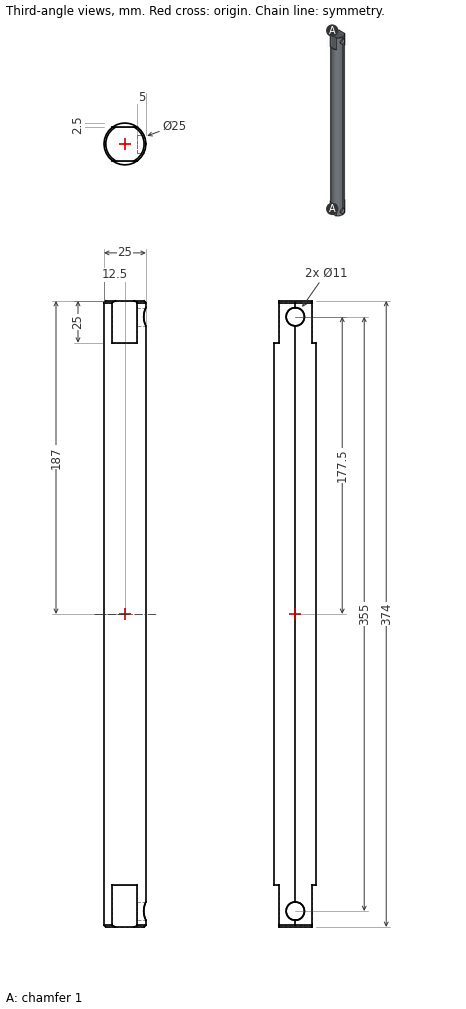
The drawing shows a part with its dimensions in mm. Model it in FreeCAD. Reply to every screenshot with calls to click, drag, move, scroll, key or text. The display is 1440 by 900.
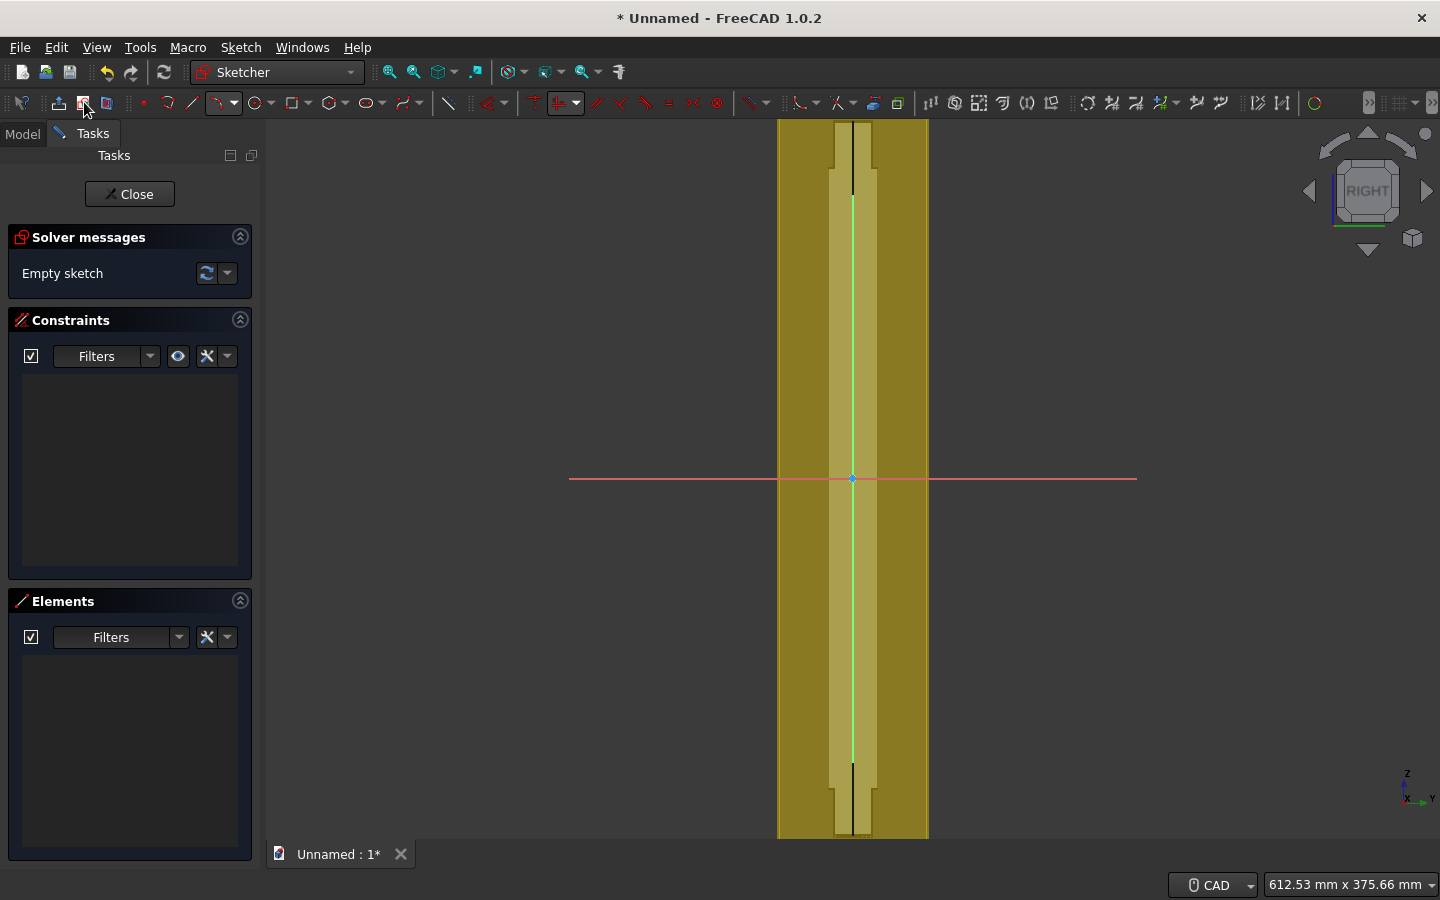
scroll(645, 479, down, 2)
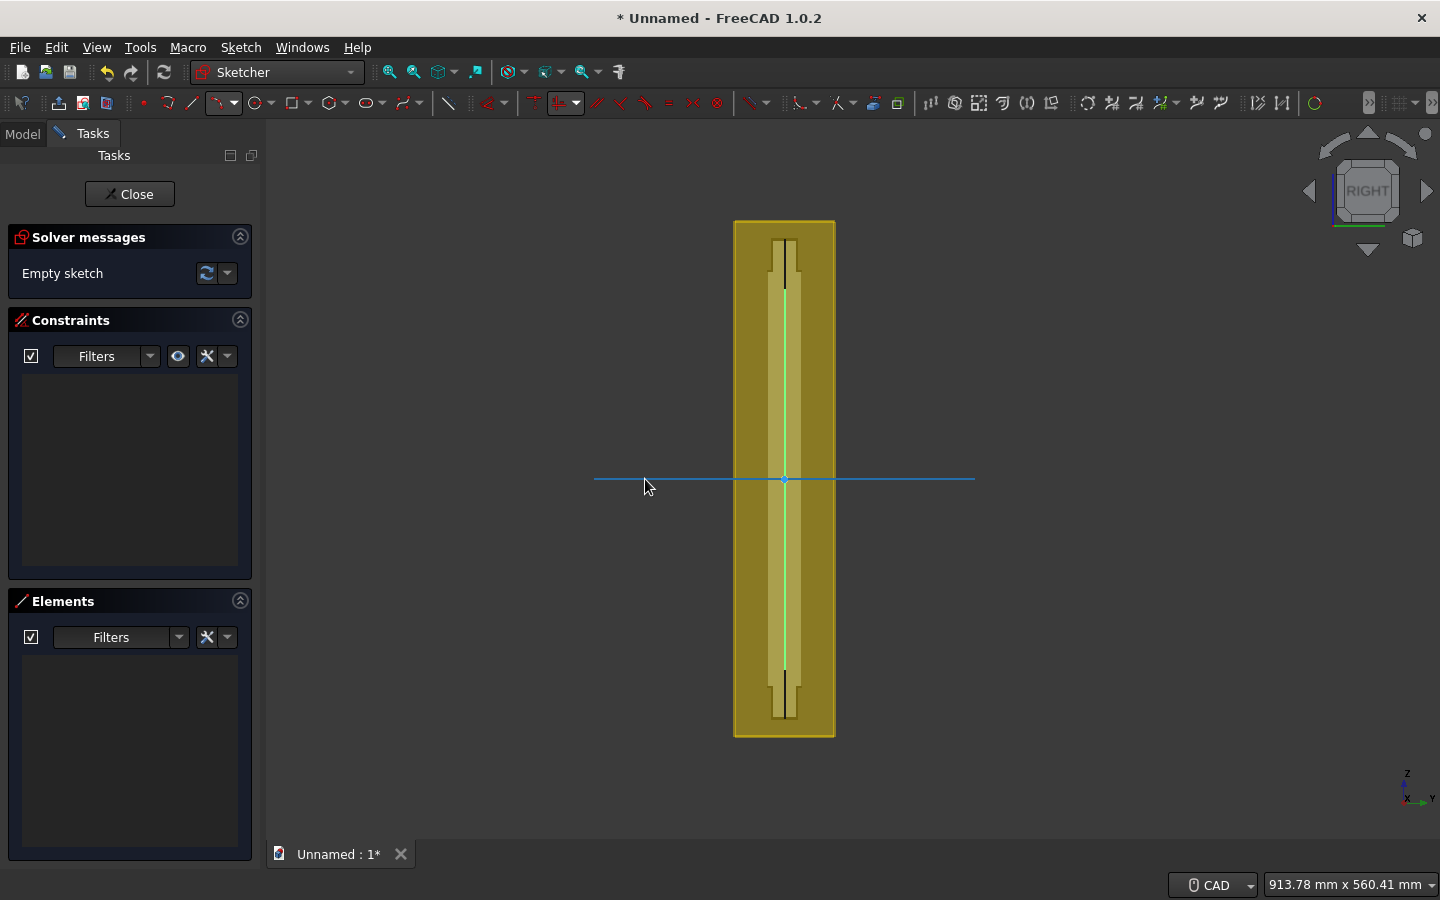
click(256, 104)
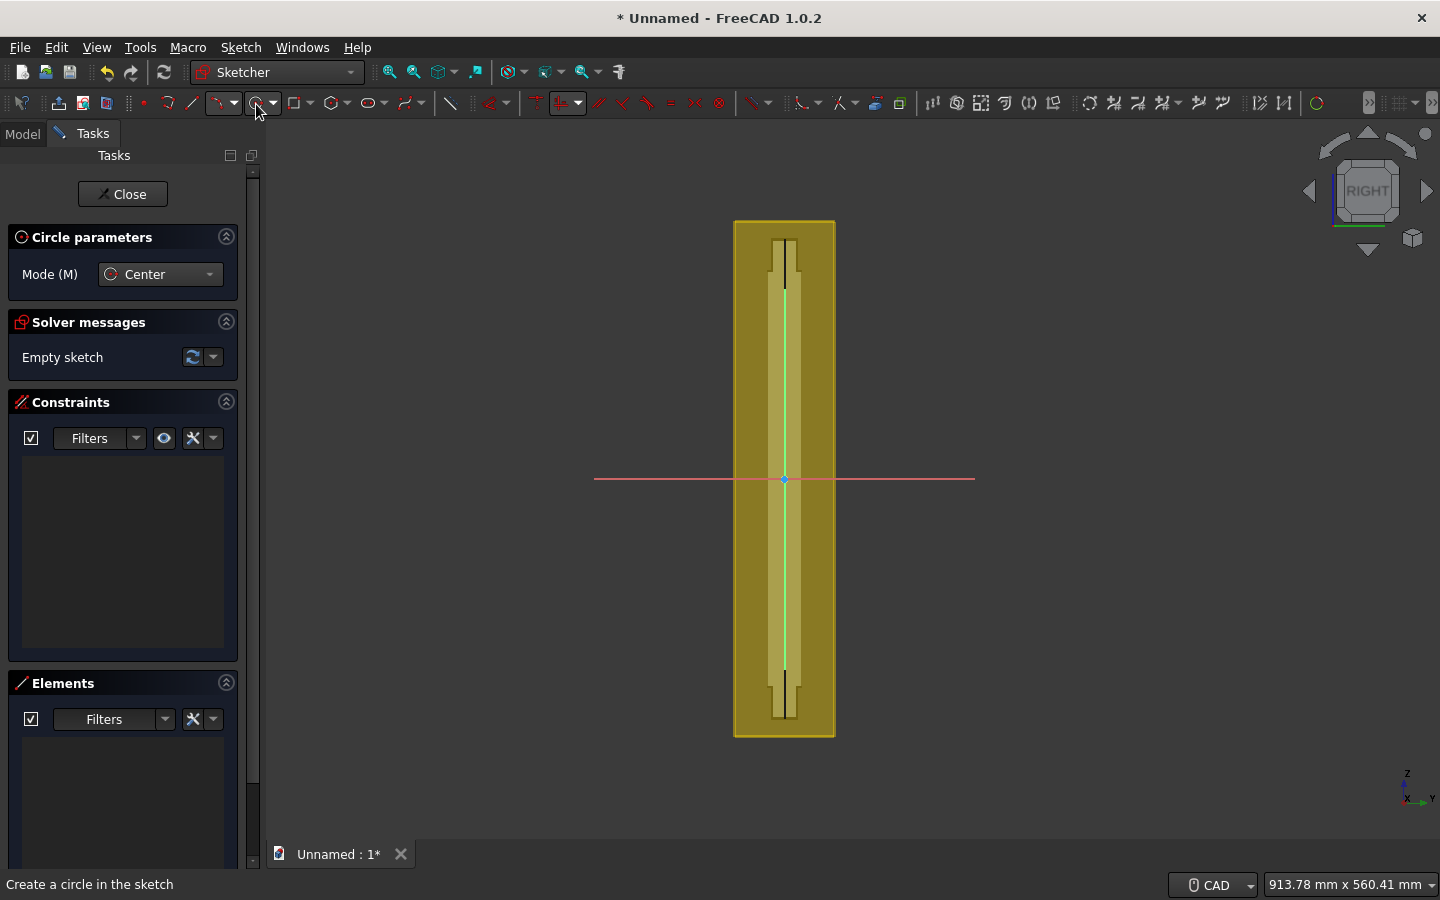
scroll(785, 251, up, 6)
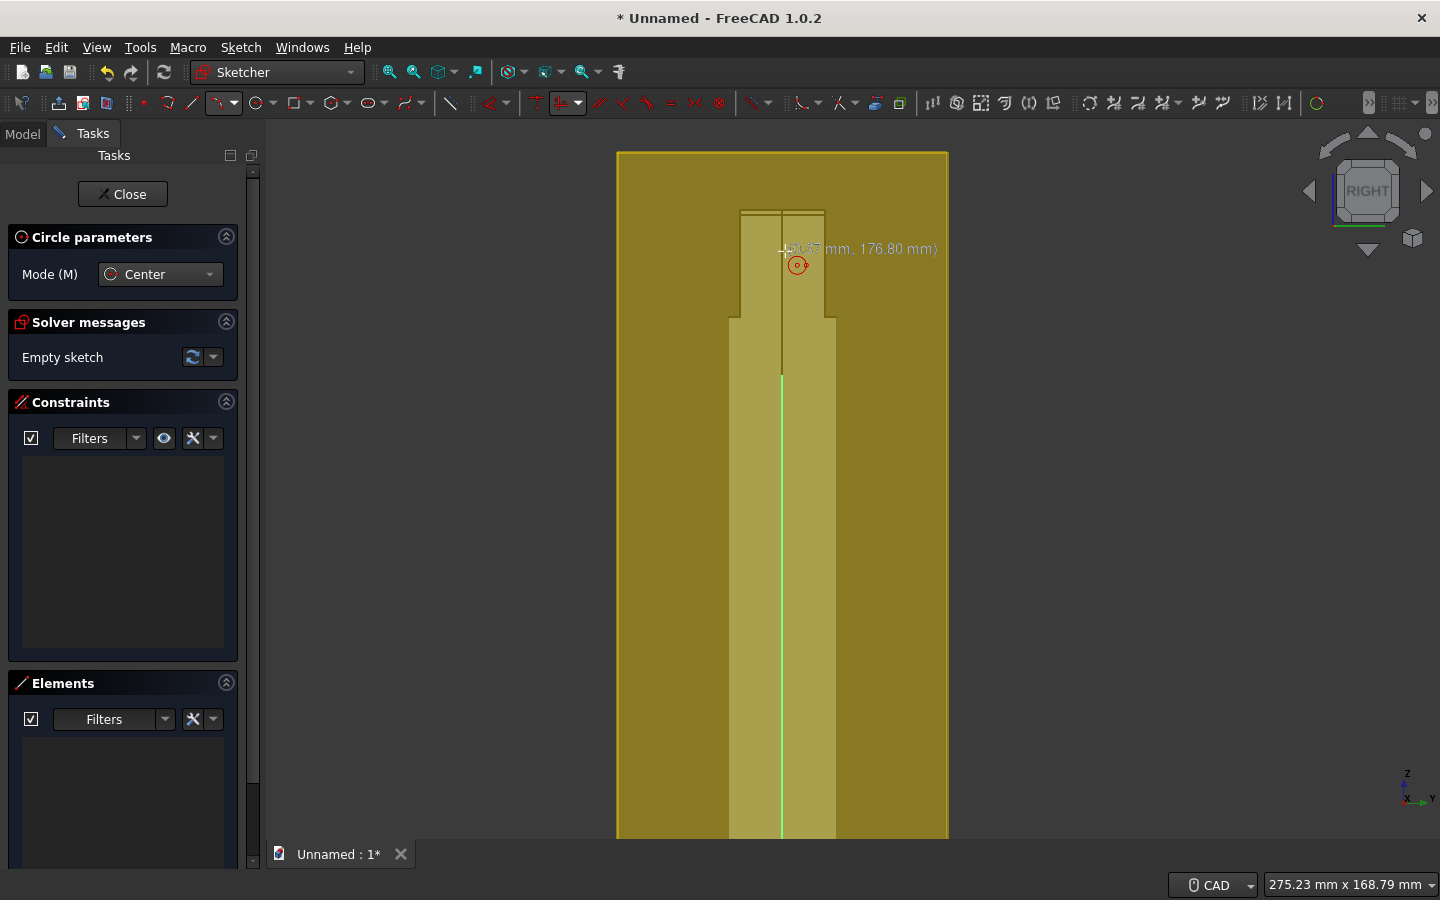
click(782, 251)
click(799, 234)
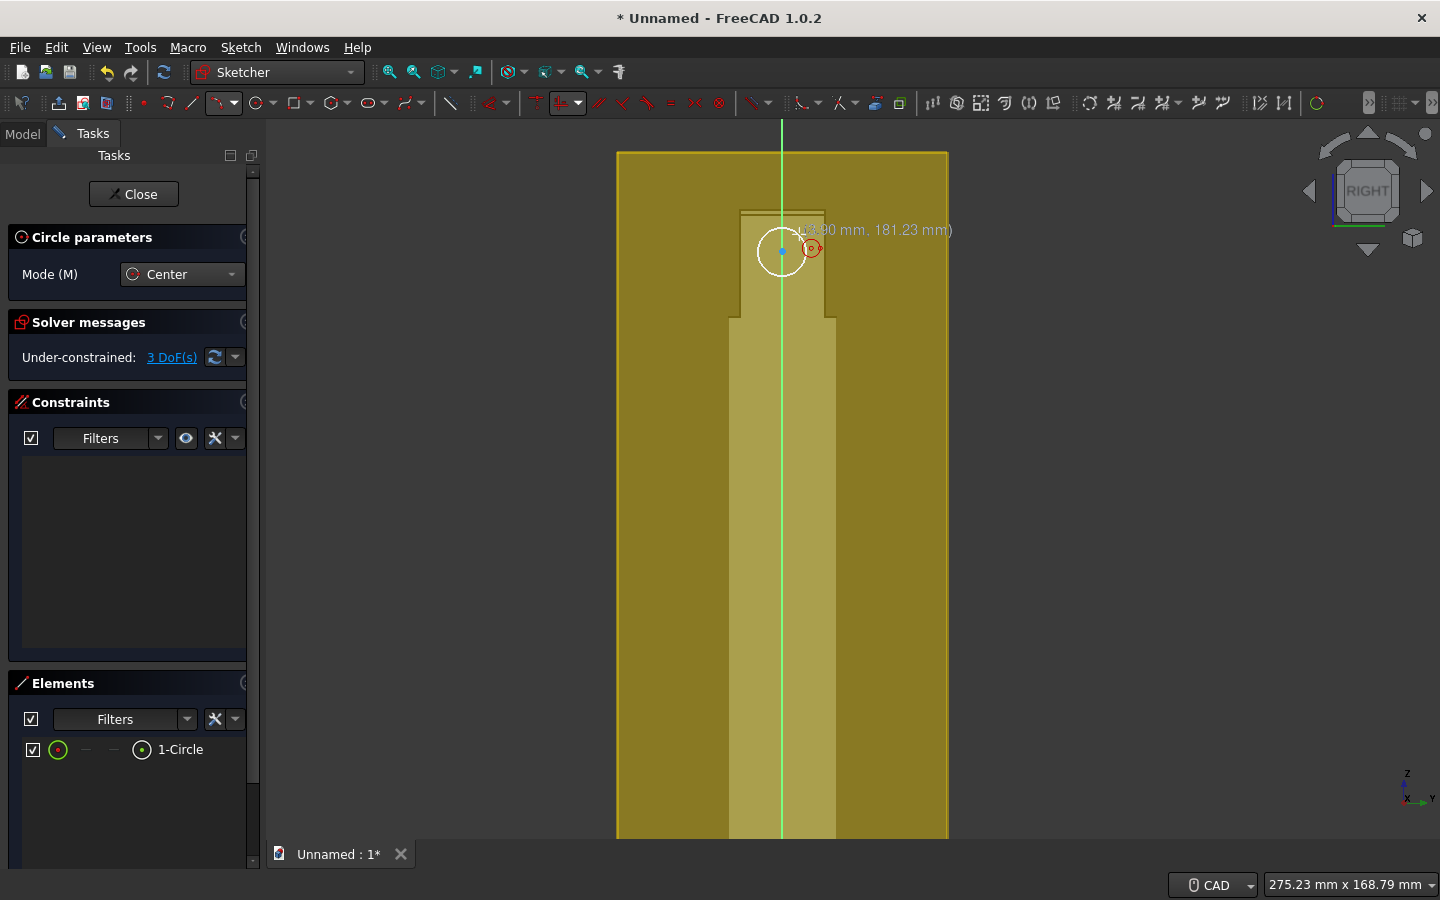
scroll(785, 251, down, 6)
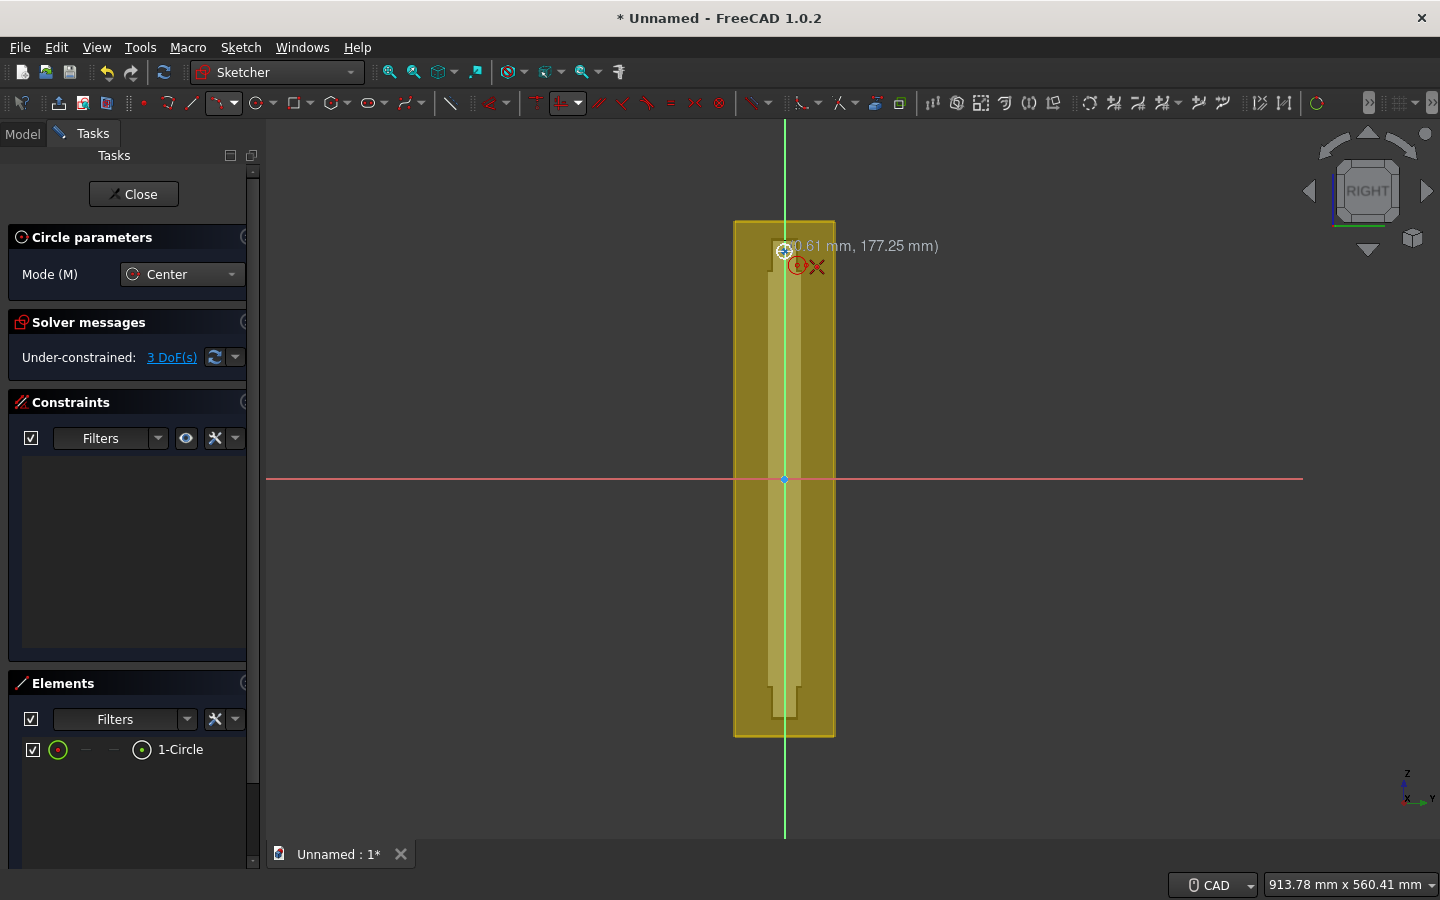
scroll(785, 707, up, 6)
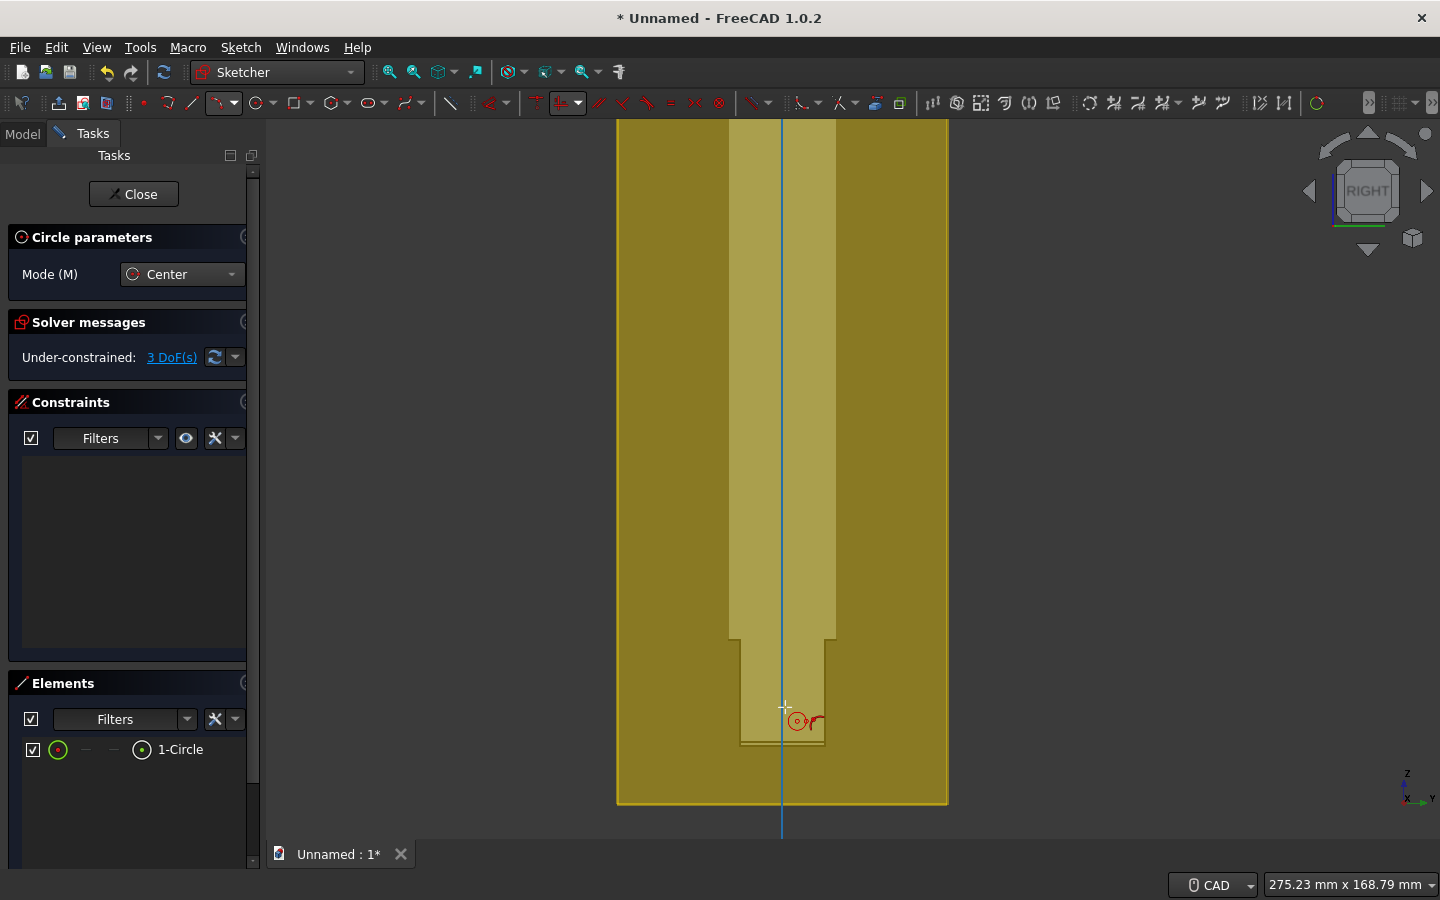
click(782, 706)
click(799, 689)
key(Escape)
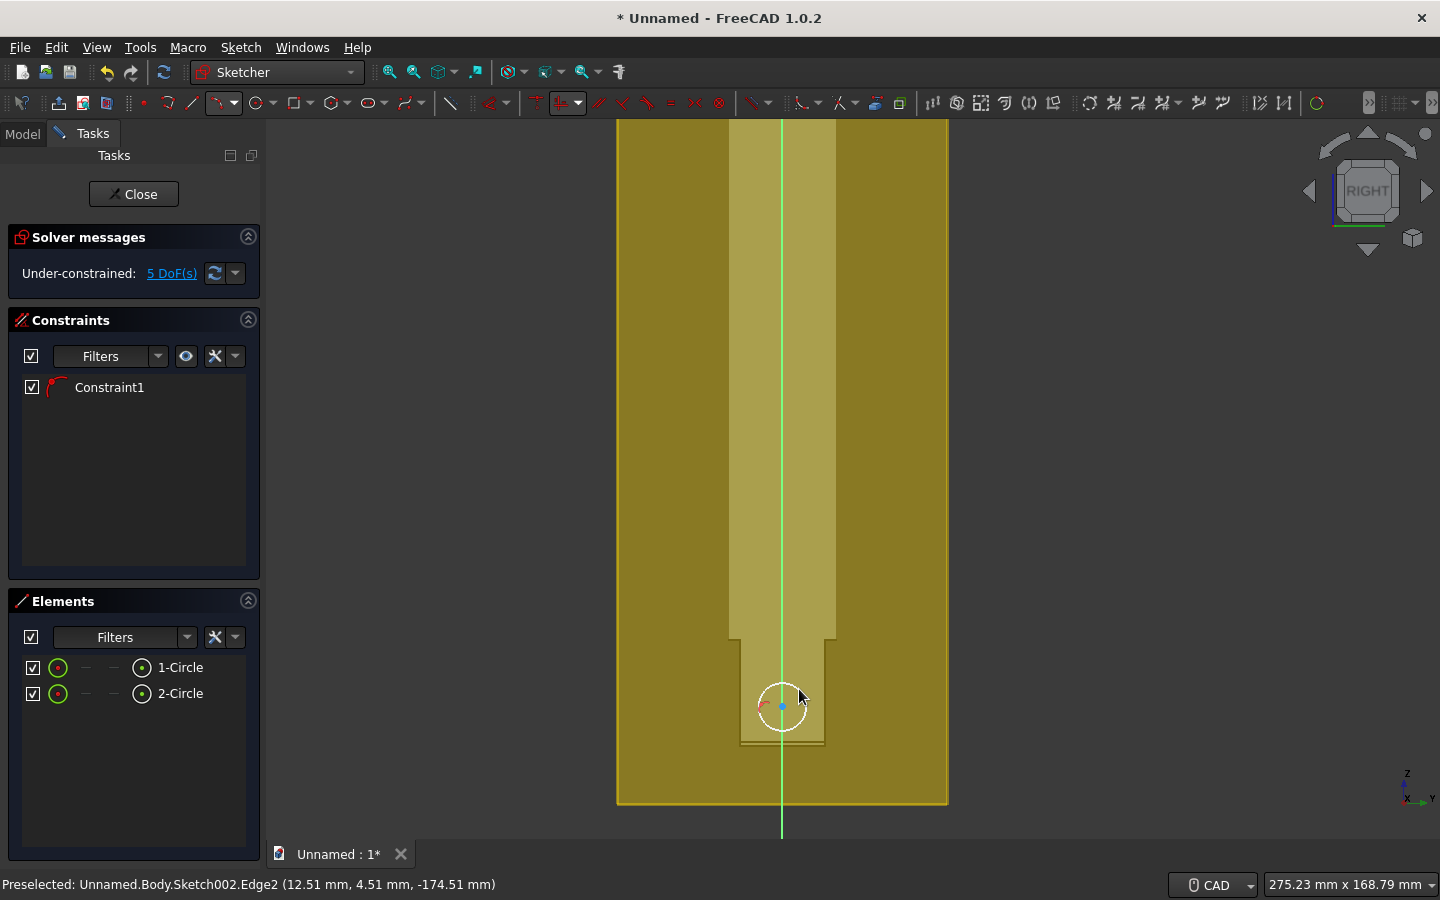
scroll(785, 708, down, 6)